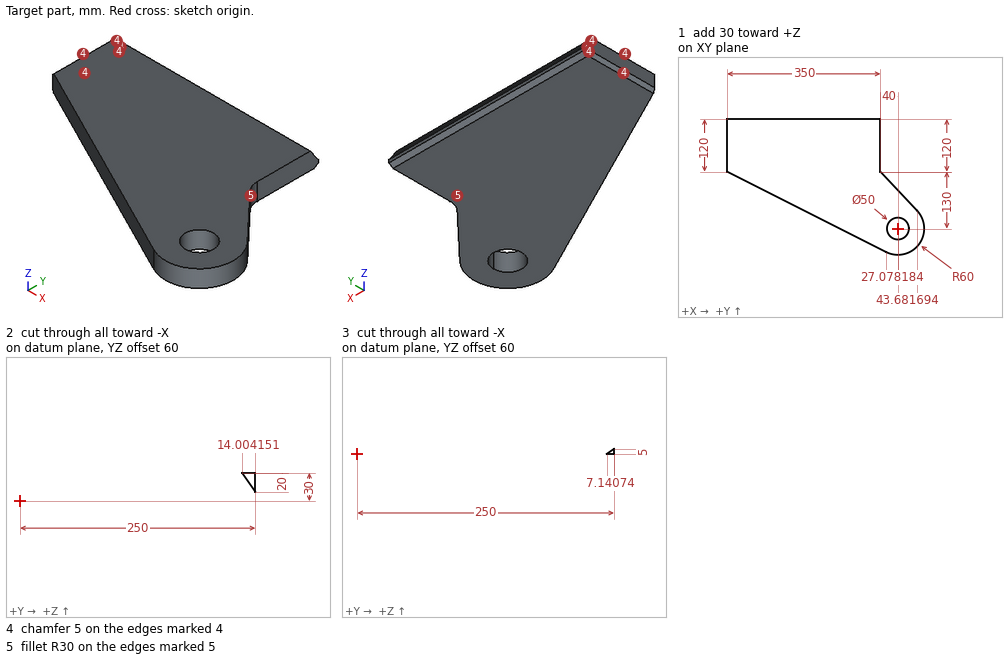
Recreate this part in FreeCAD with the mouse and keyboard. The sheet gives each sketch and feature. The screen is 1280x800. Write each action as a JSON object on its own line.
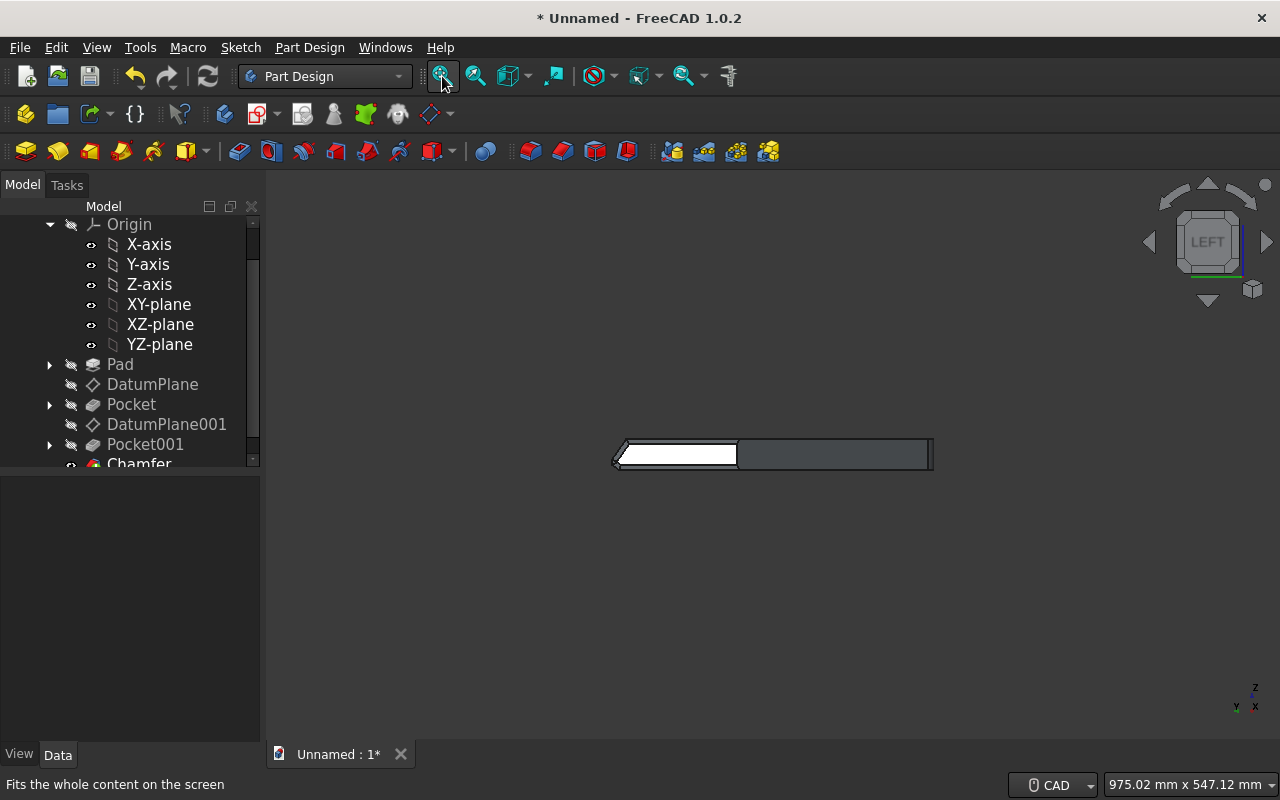
{"action": "left_click", "coordinate": [444, 76]}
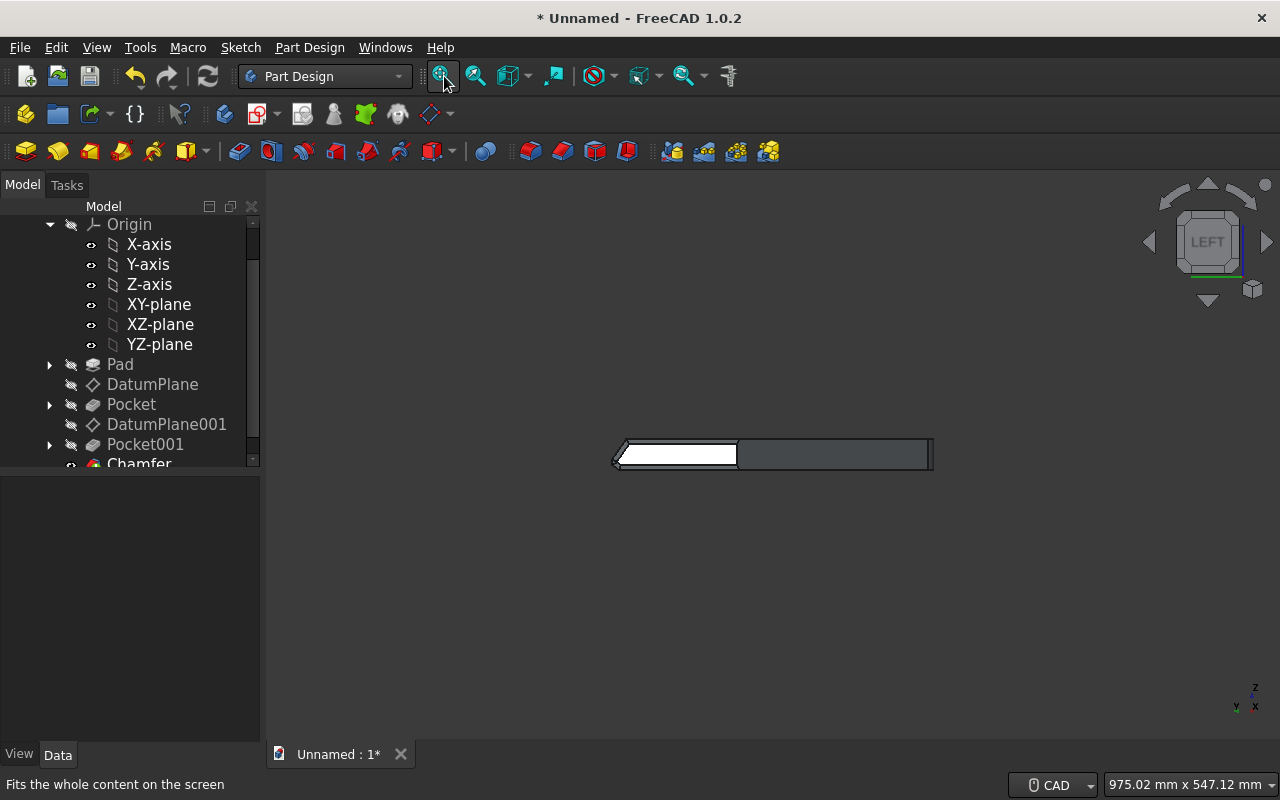
{"action": "key", "text": "v 3"}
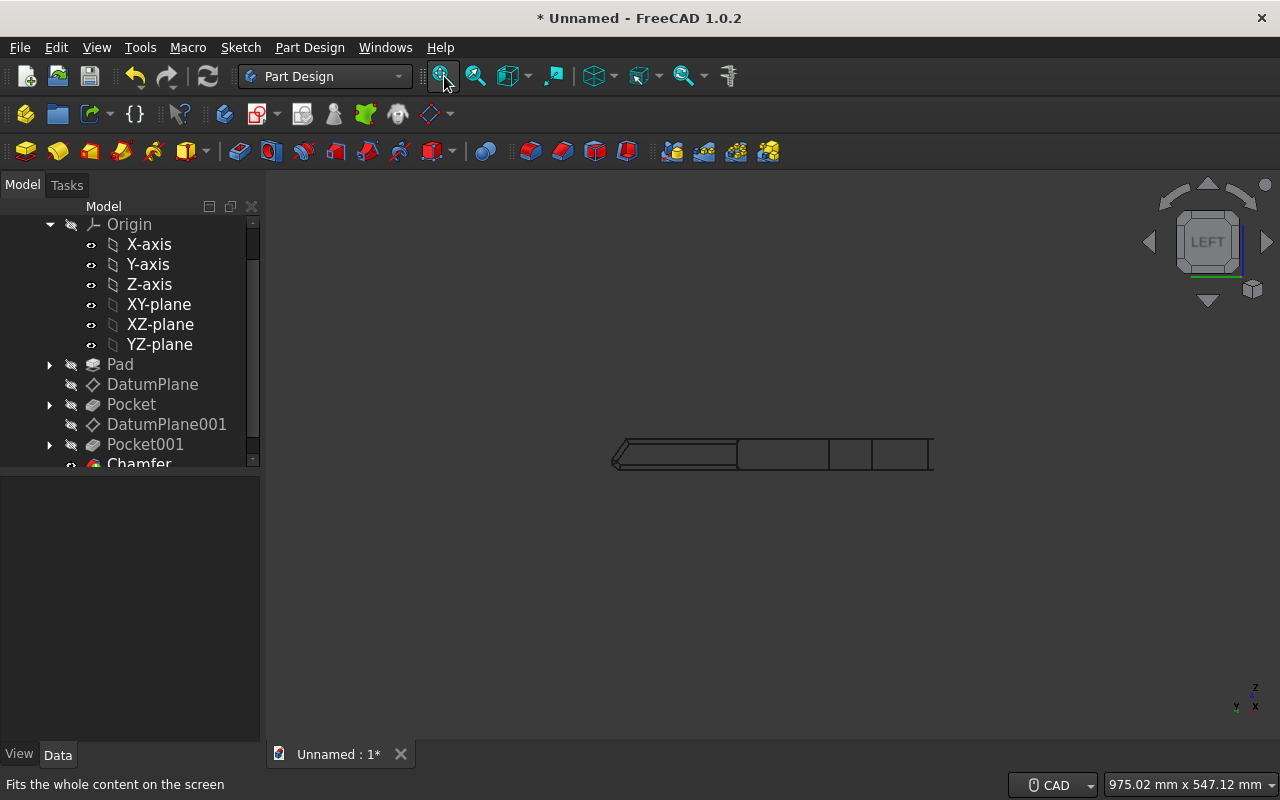
{"action": "key", "text": "0"}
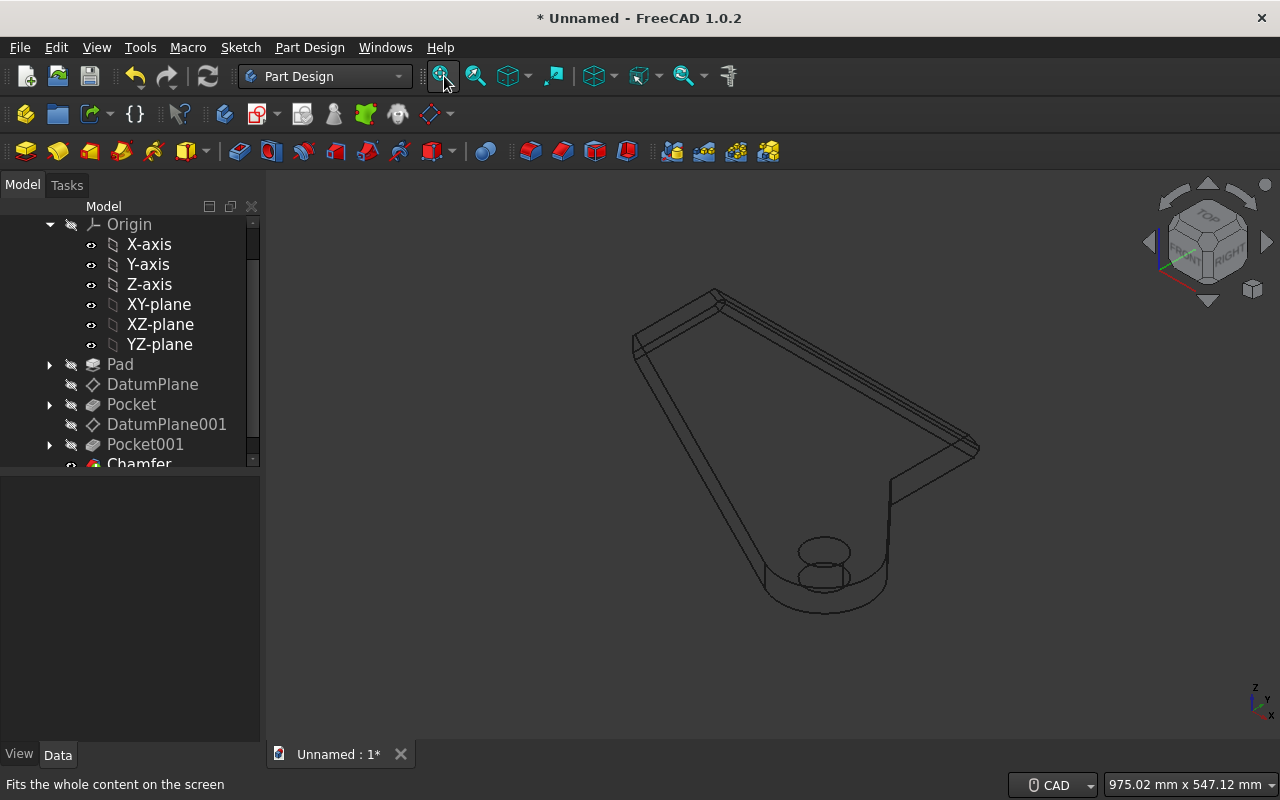
{"action": "scroll", "coordinate": [891, 492], "scroll_direction": "up", "scroll_amount": 6}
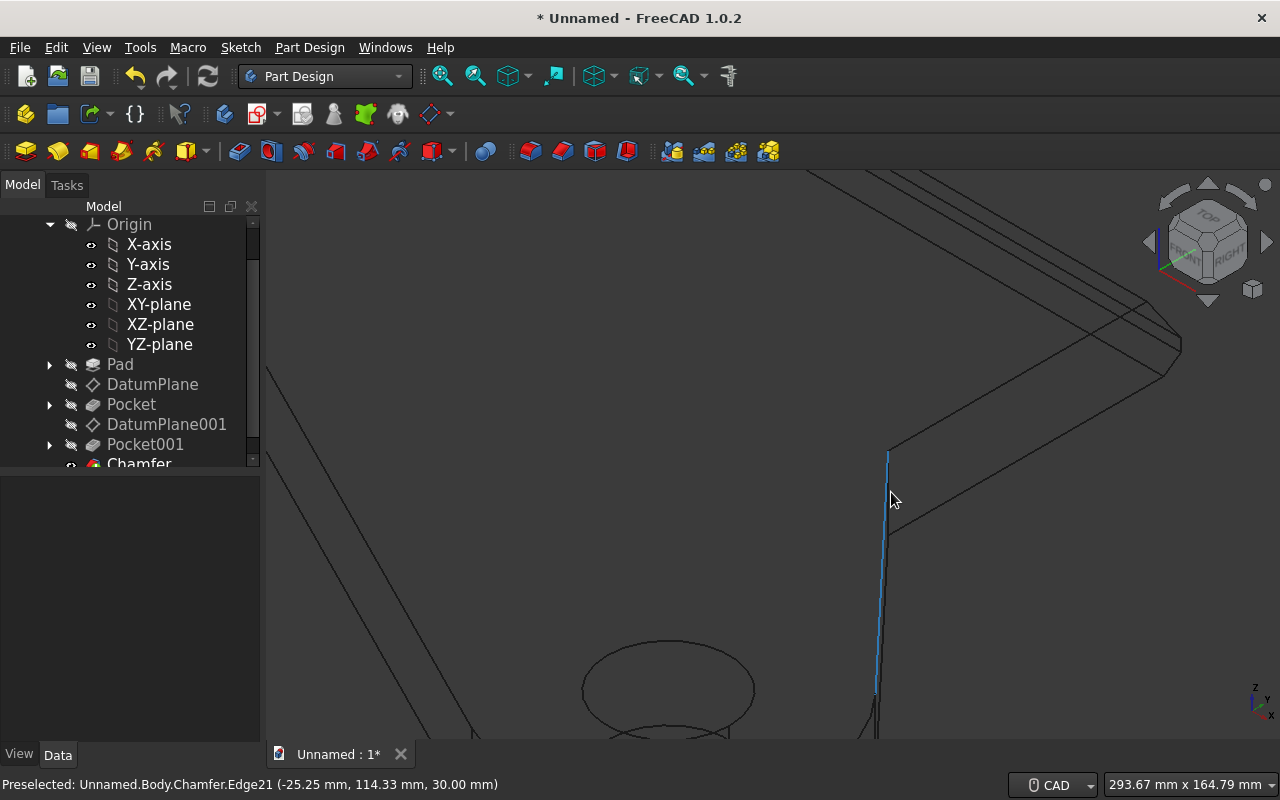
{"action": "key", "text": "v f"}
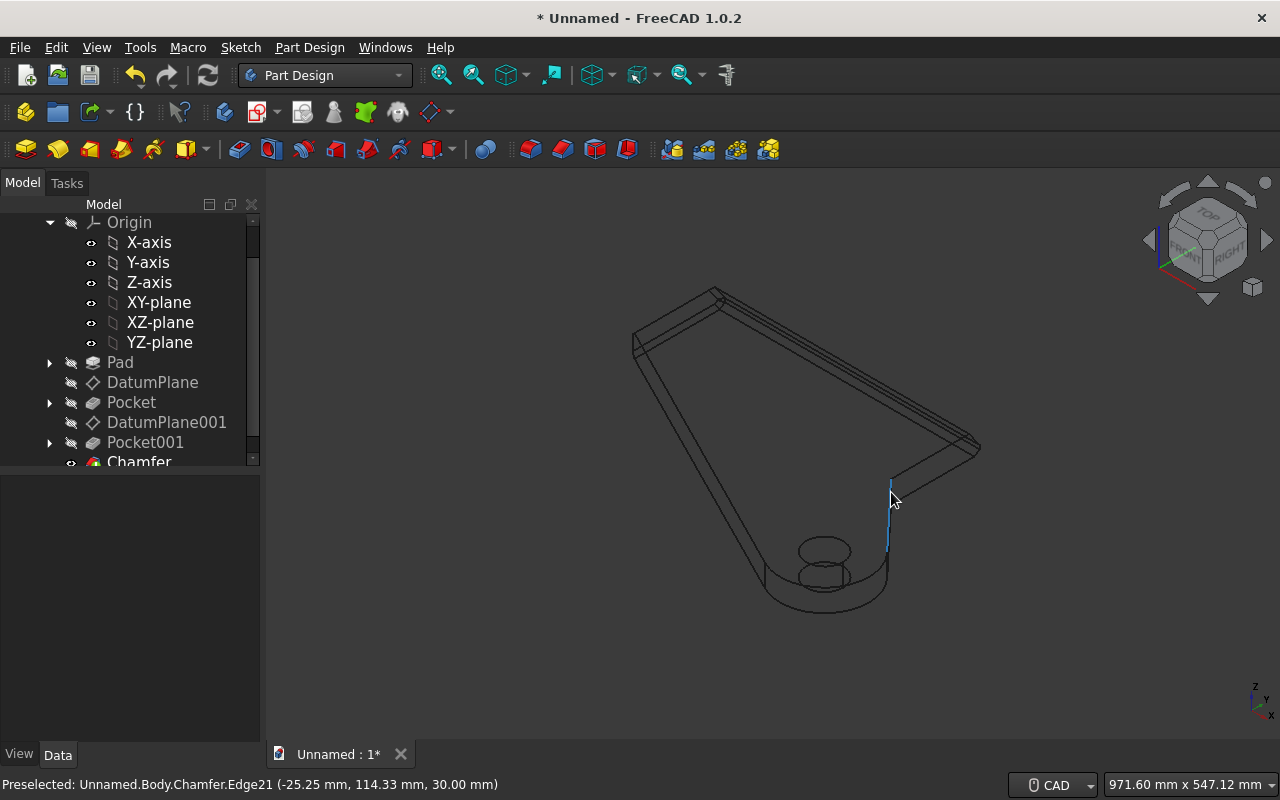
{"action": "key", "text": "2"}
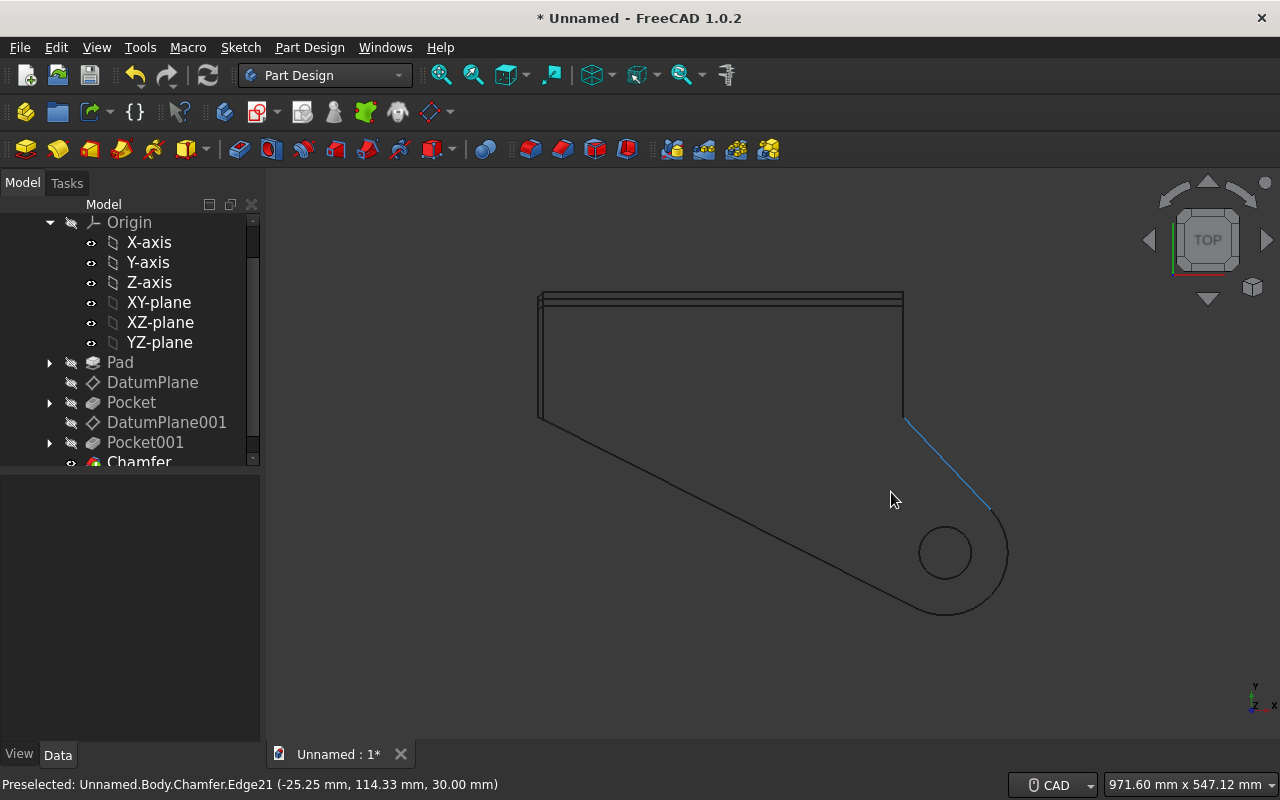
{"action": "scroll", "coordinate": [903, 416], "scroll_direction": "up", "scroll_amount": 6}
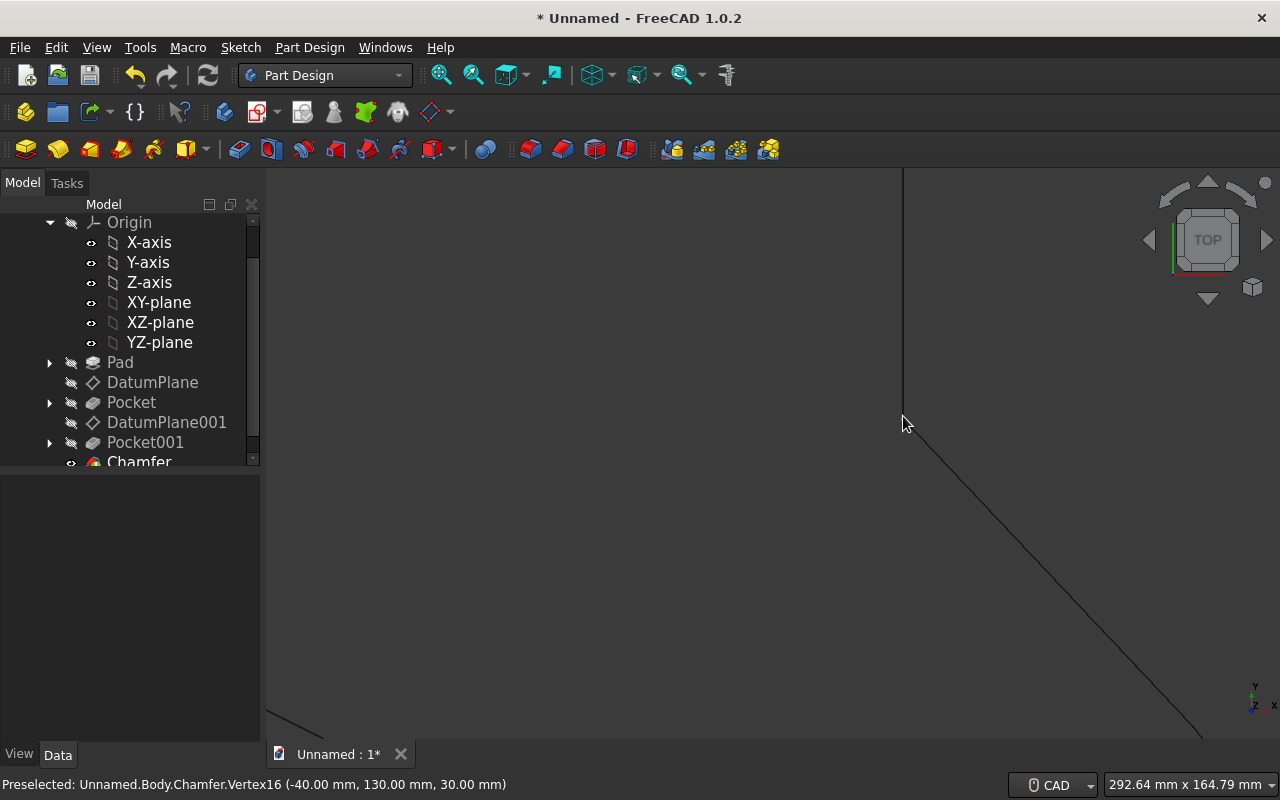
{"action": "key", "text": "v f"}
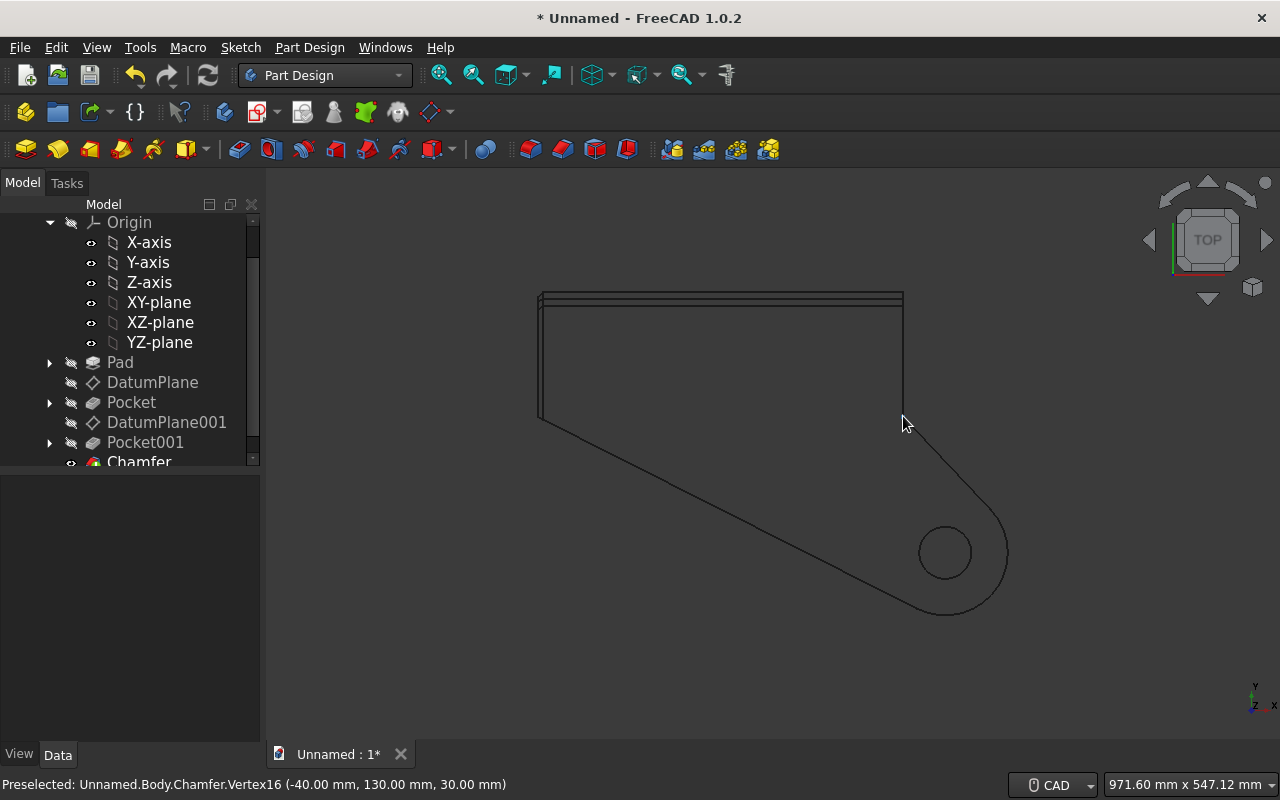
{"action": "key", "text": "1"}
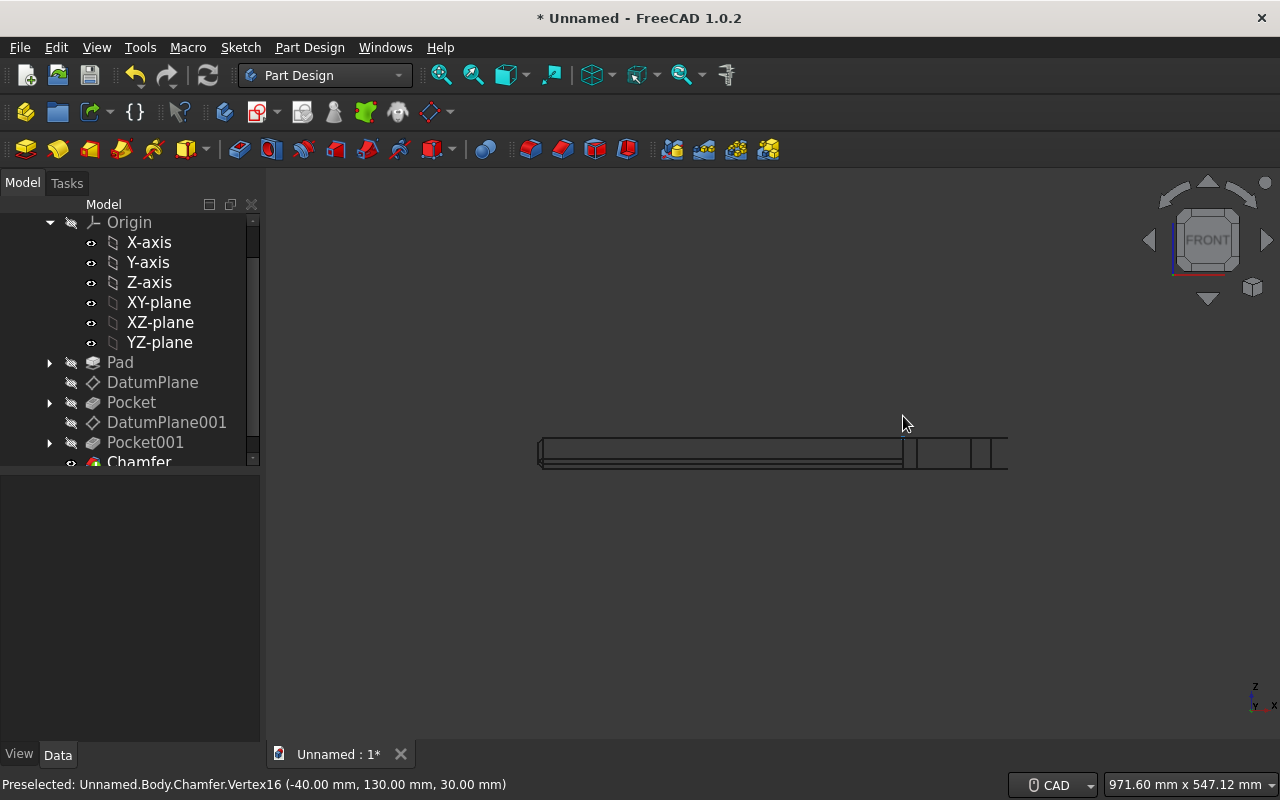
{"action": "left_click", "coordinate": [903, 452]}